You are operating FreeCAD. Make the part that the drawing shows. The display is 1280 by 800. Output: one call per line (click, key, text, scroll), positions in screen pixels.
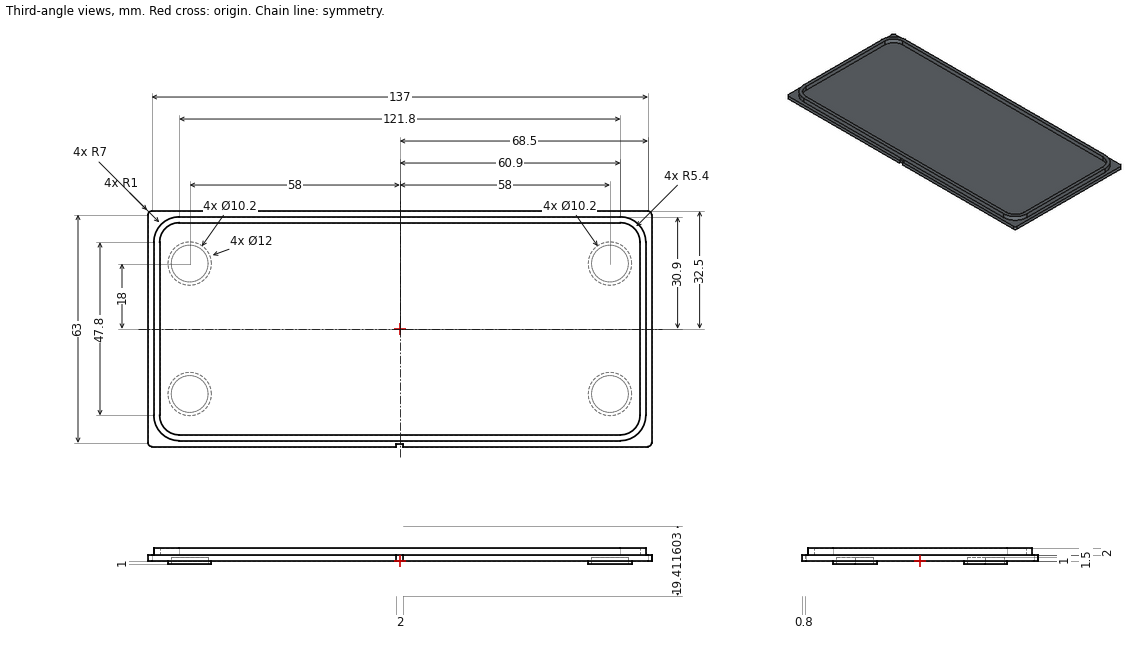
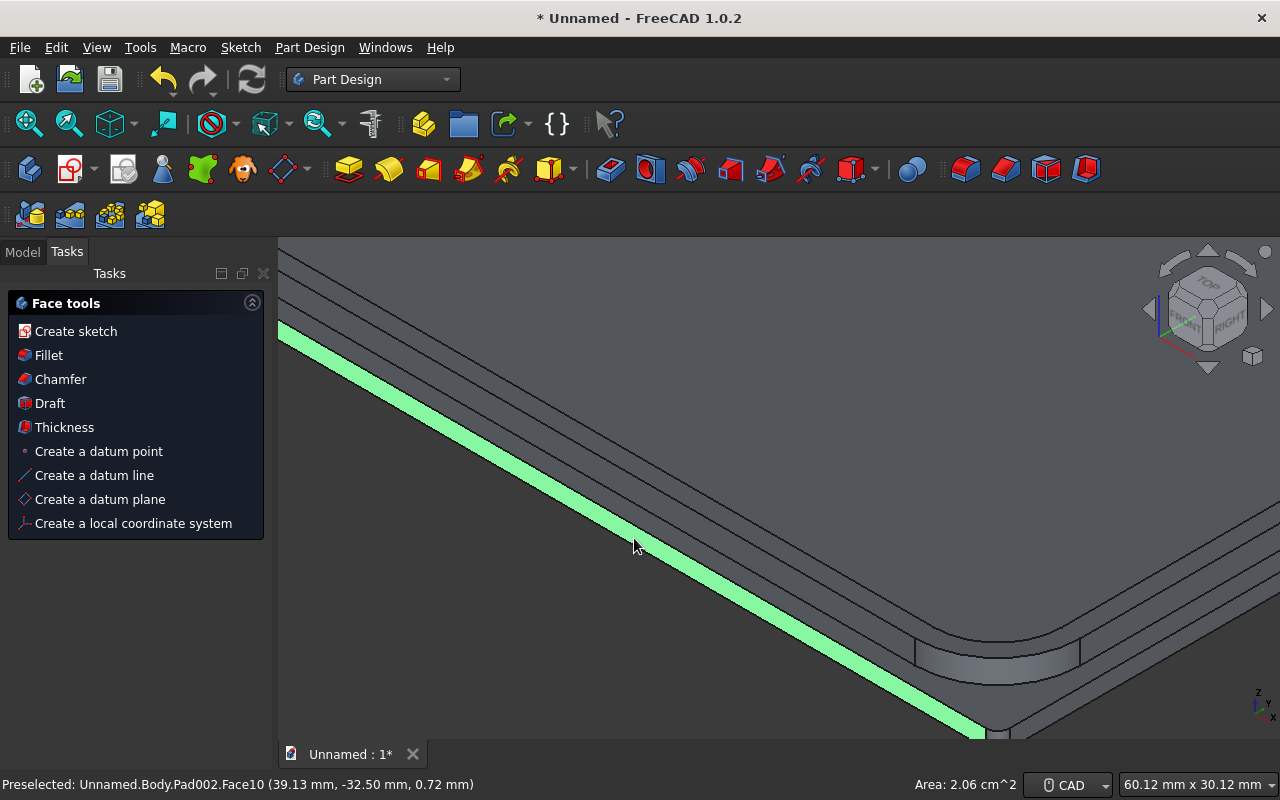
click(70, 170)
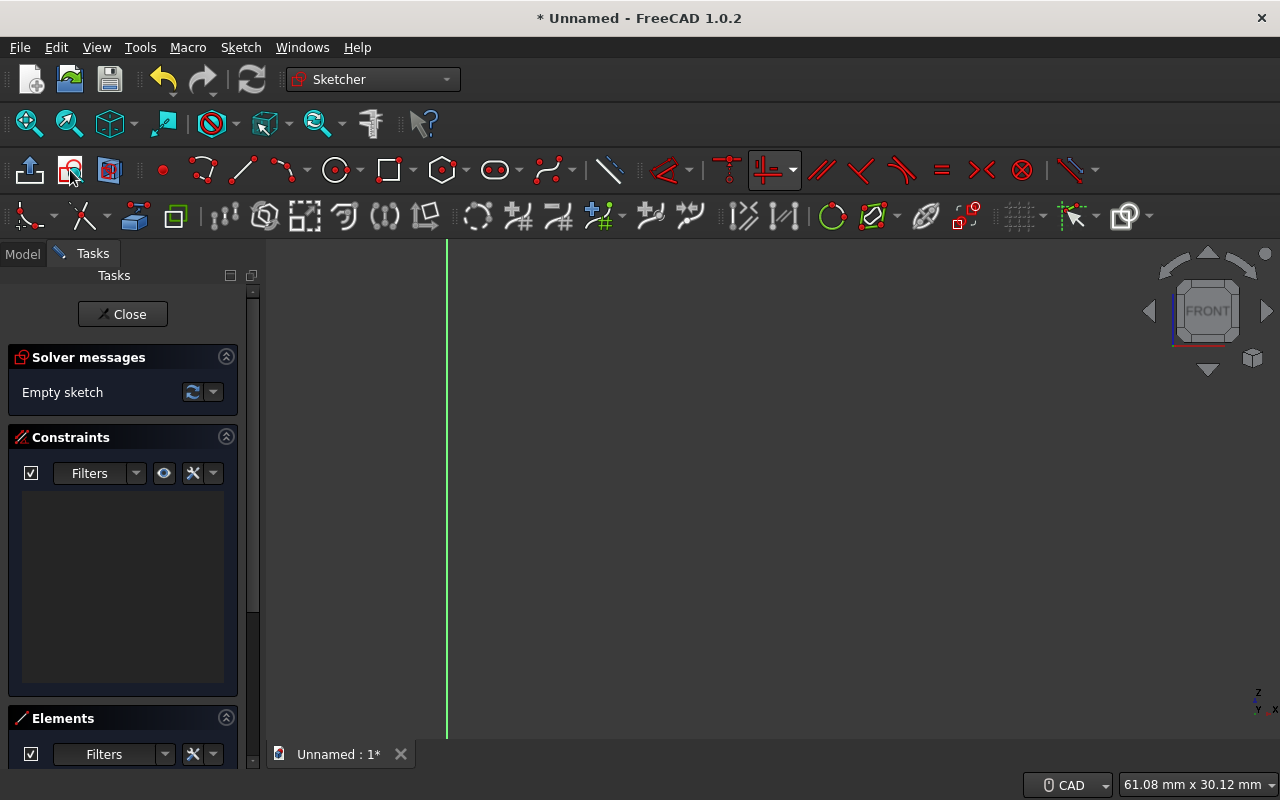
scroll(1018, 711, down, 3)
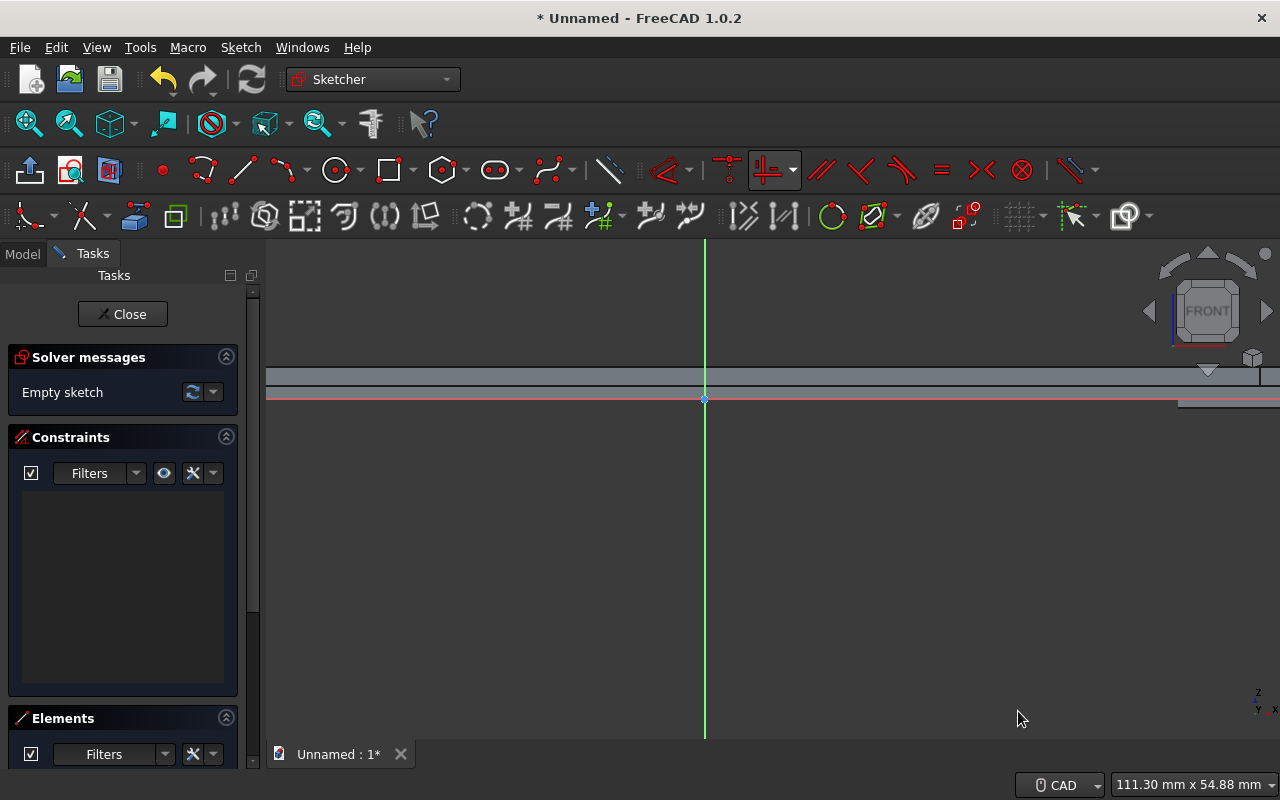
scroll(705, 290, up, 3)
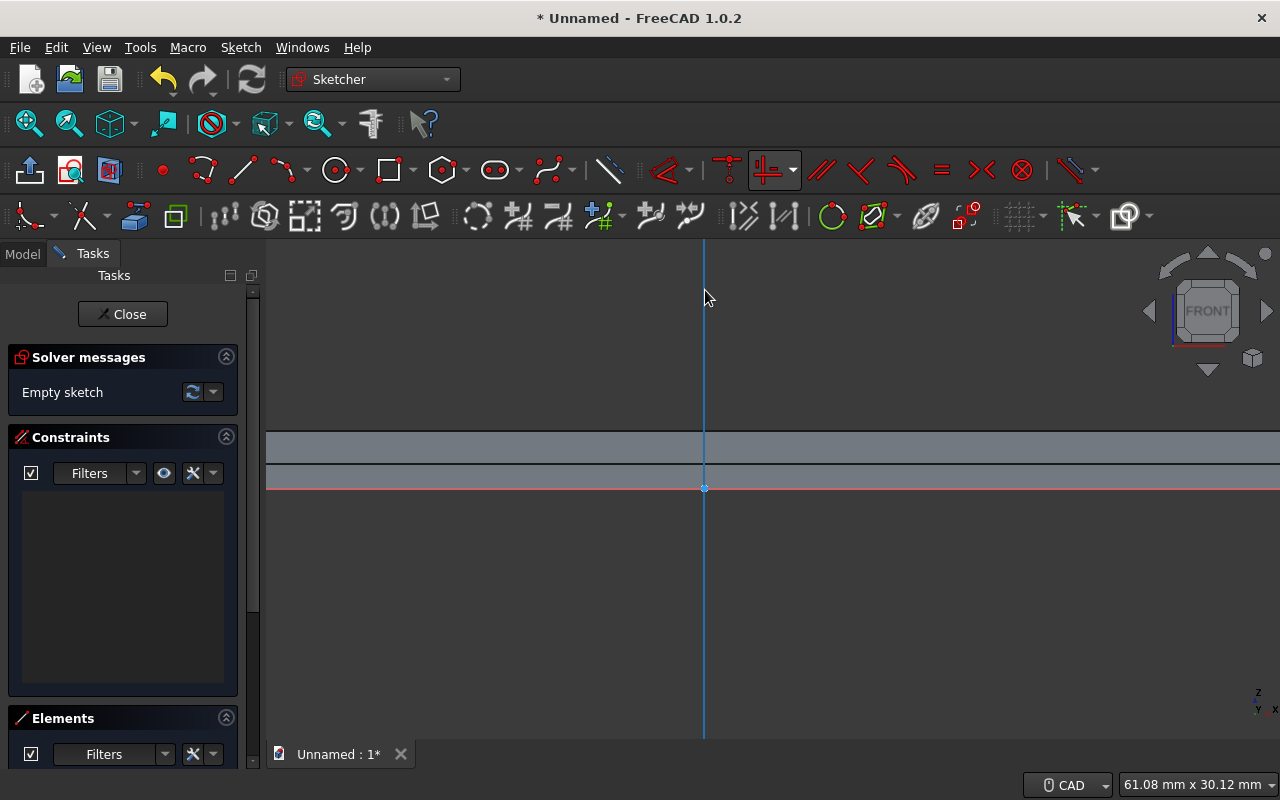
key(g)
key(v)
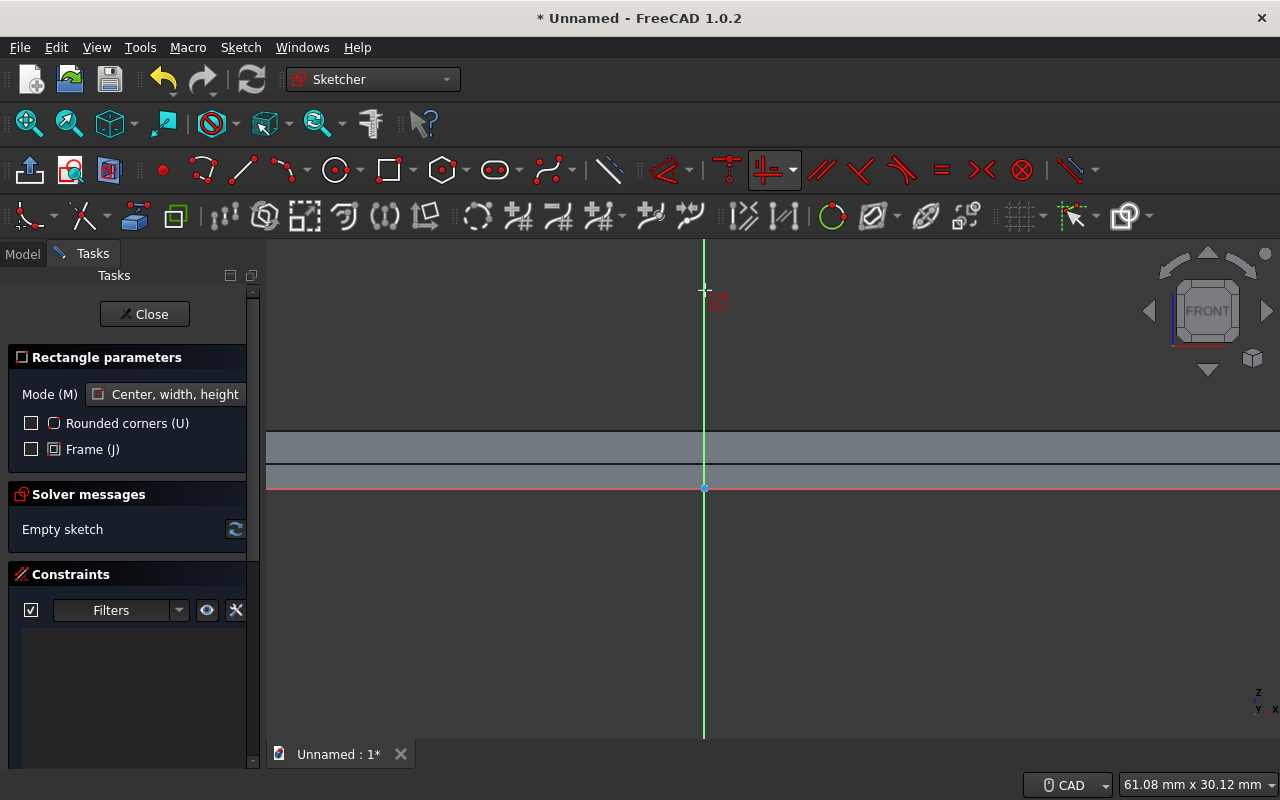
click(704, 489)
move(721, 328)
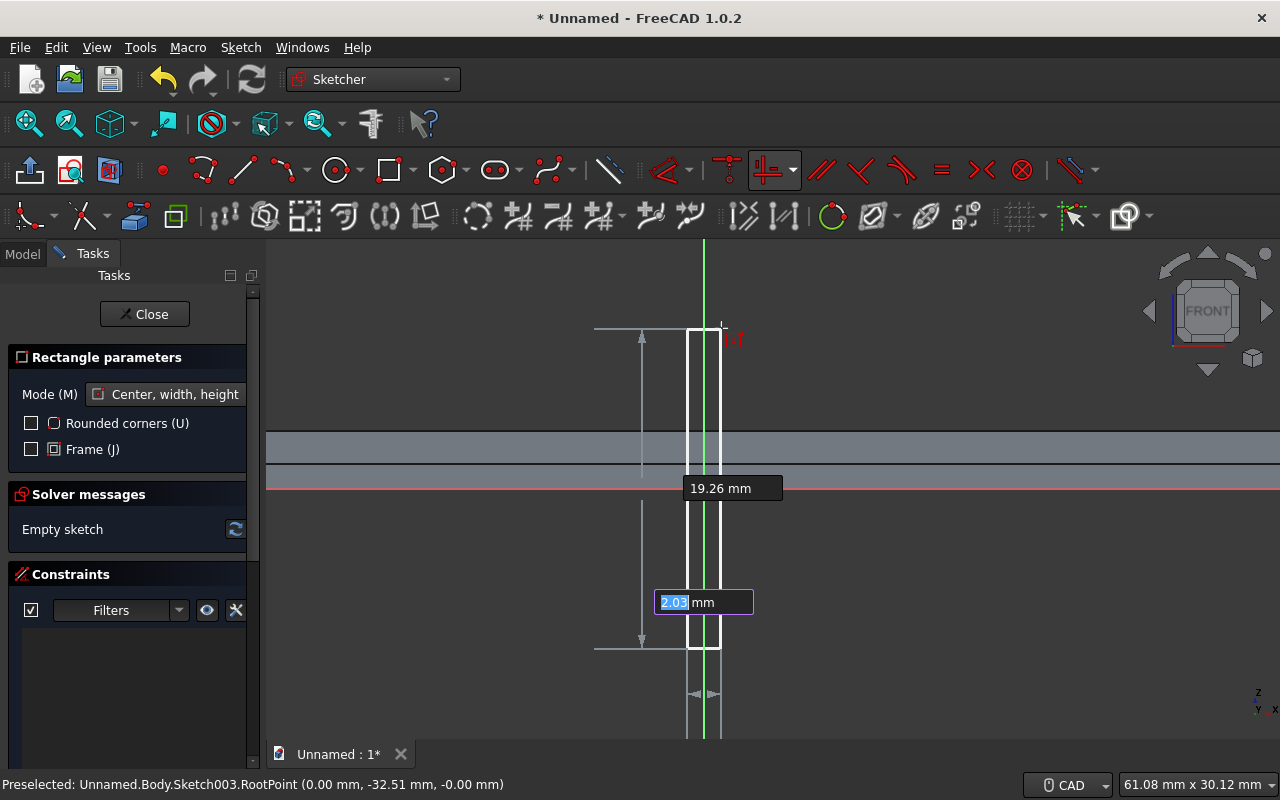
text(2)
key(Tab)
text(19.411603)
key(Return)
key(Escape)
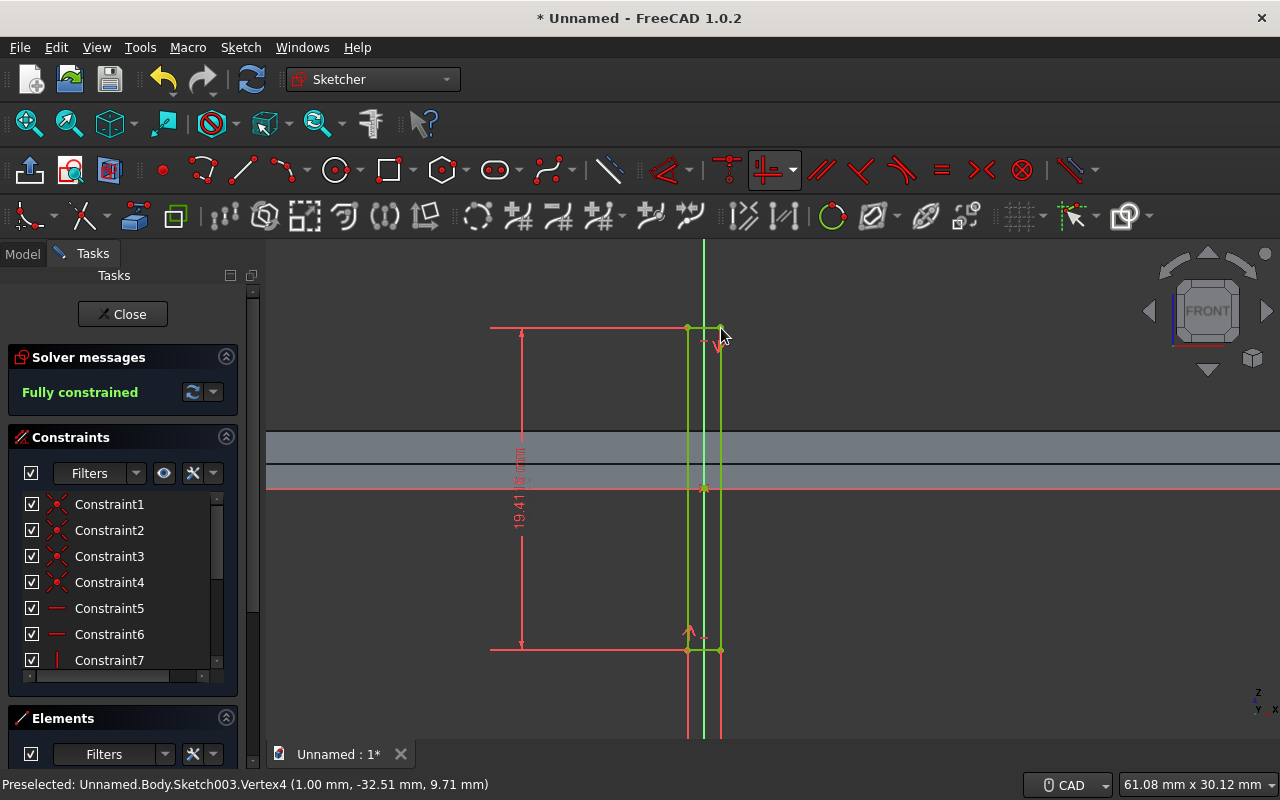
click(123, 314)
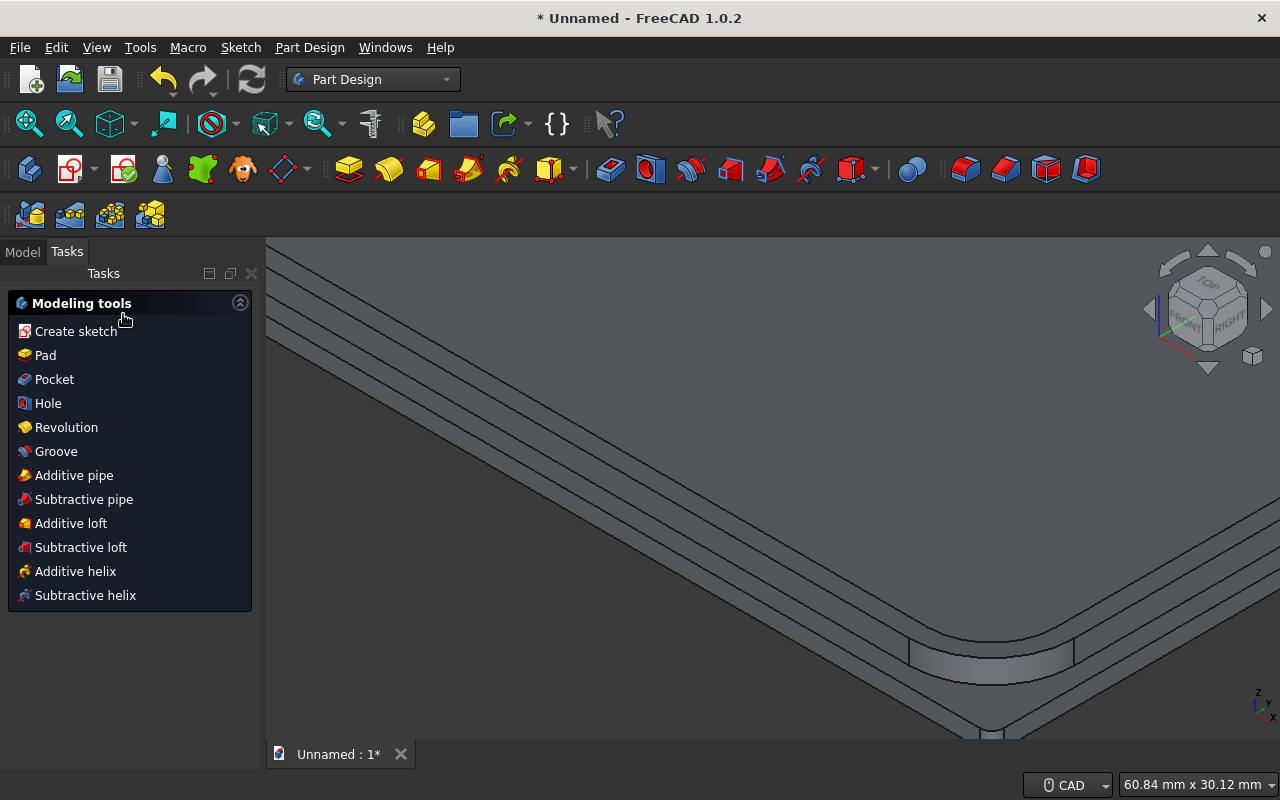
click(612, 170)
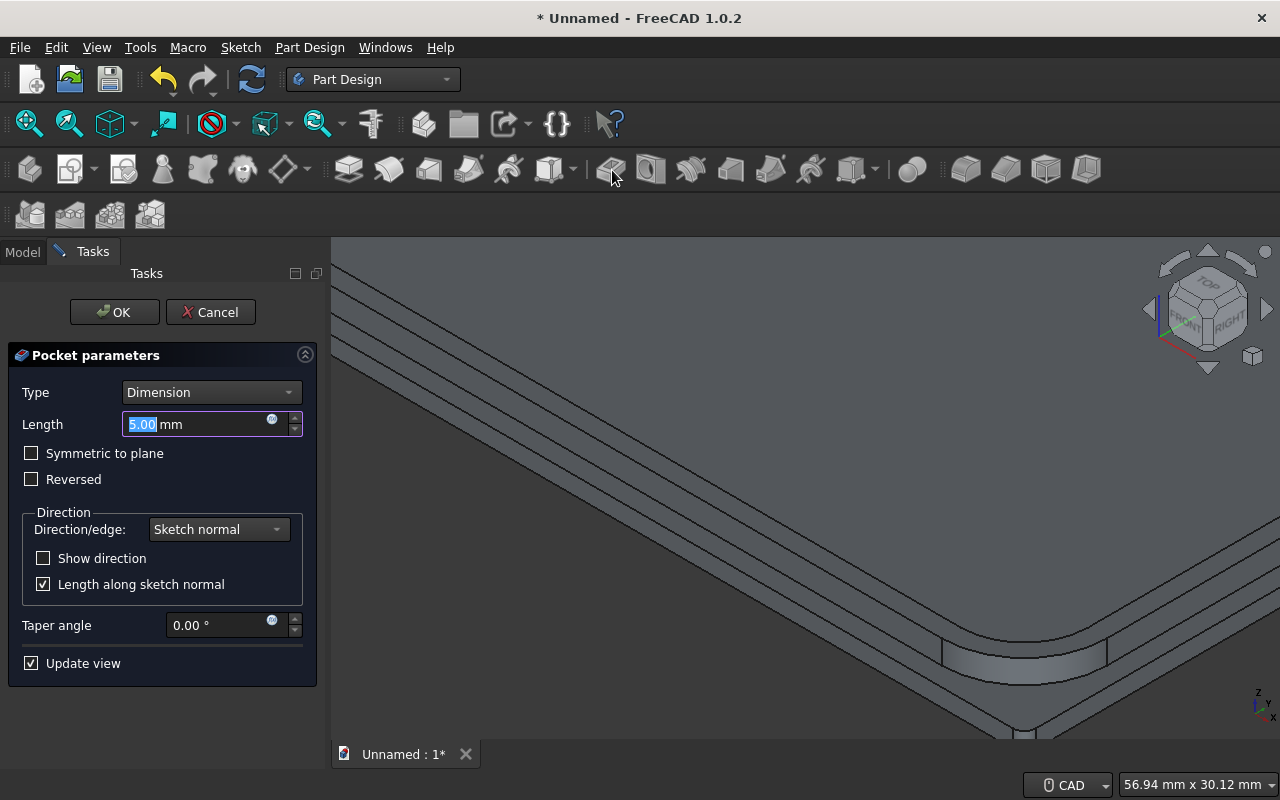
text(0.8)
key(Tab)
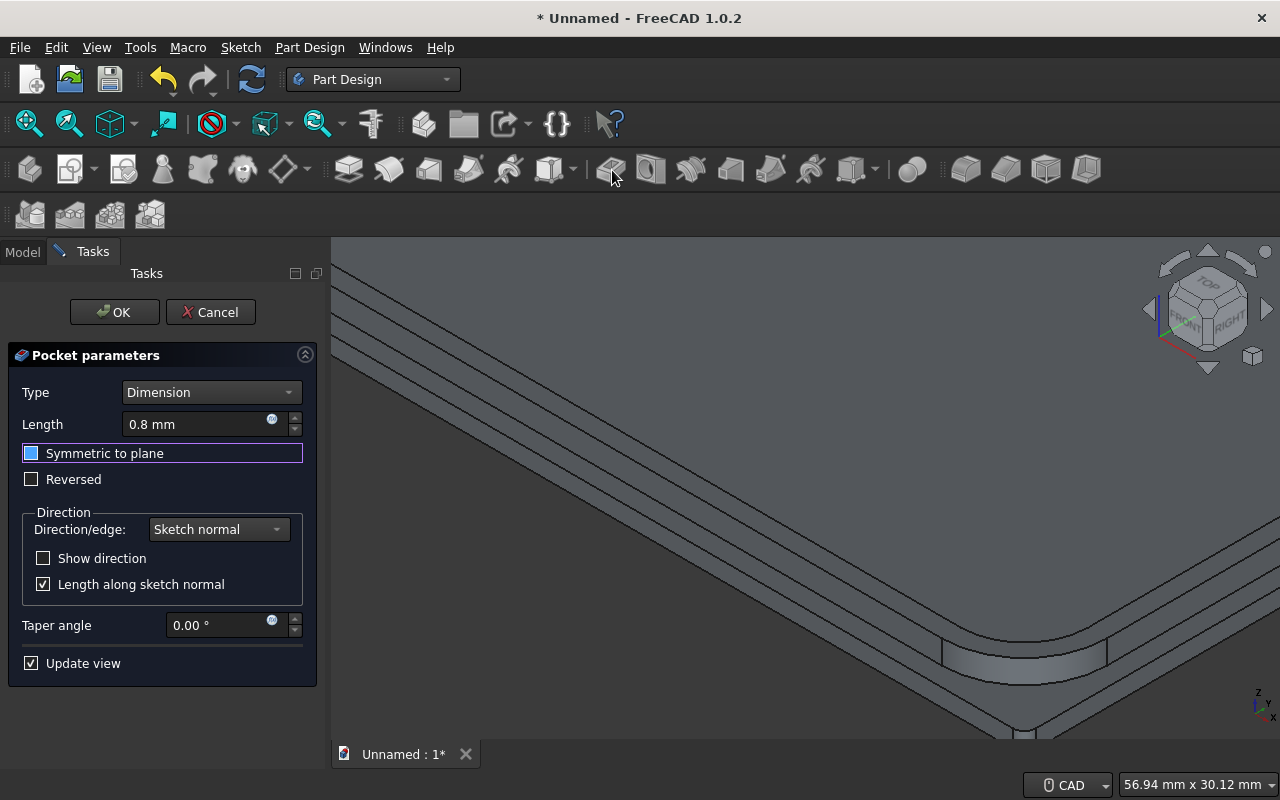
click(115, 312)